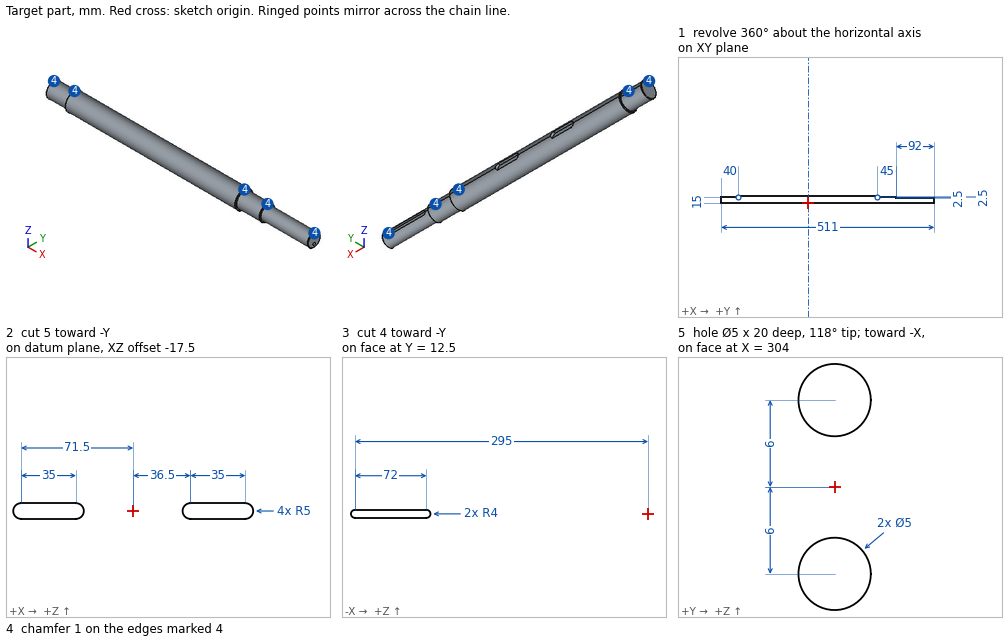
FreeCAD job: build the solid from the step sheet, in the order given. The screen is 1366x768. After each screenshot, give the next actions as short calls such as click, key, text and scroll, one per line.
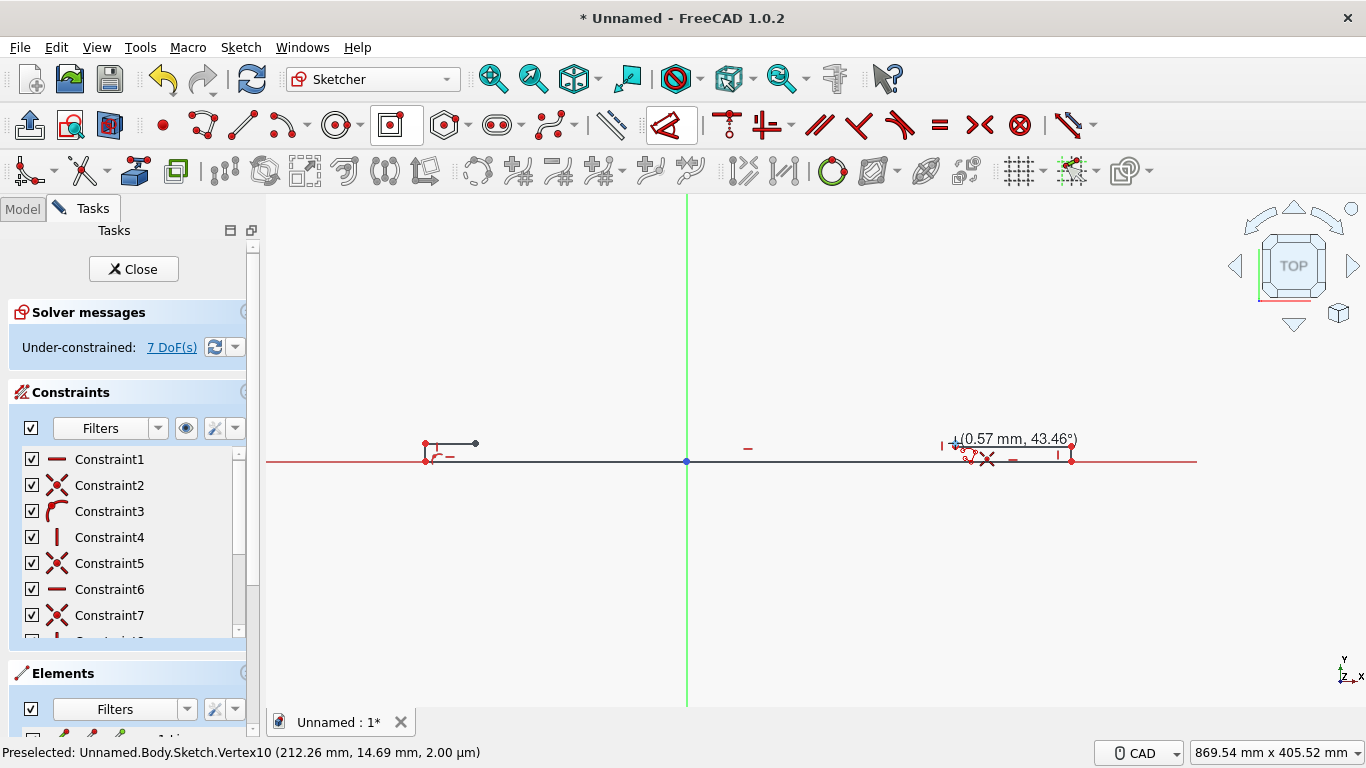
click(898, 443)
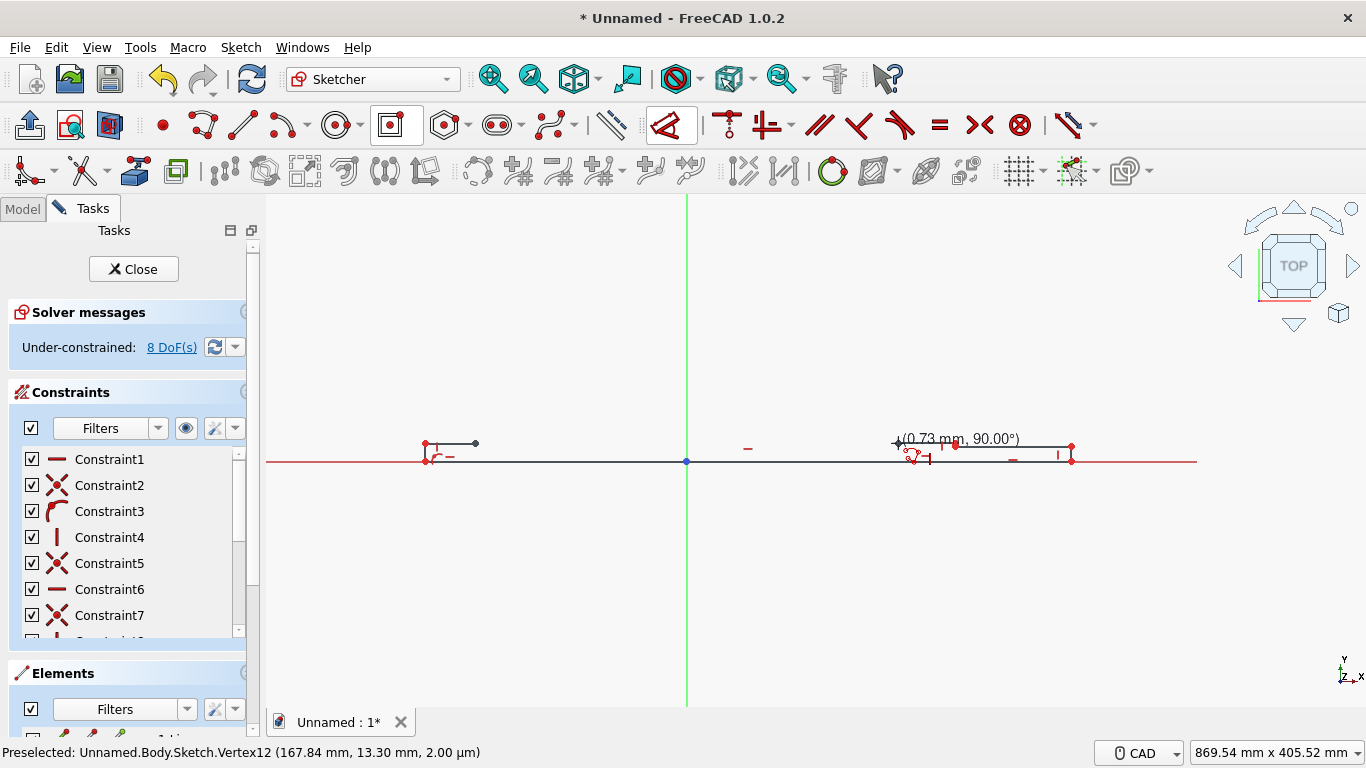
scroll(898, 440, up, 9)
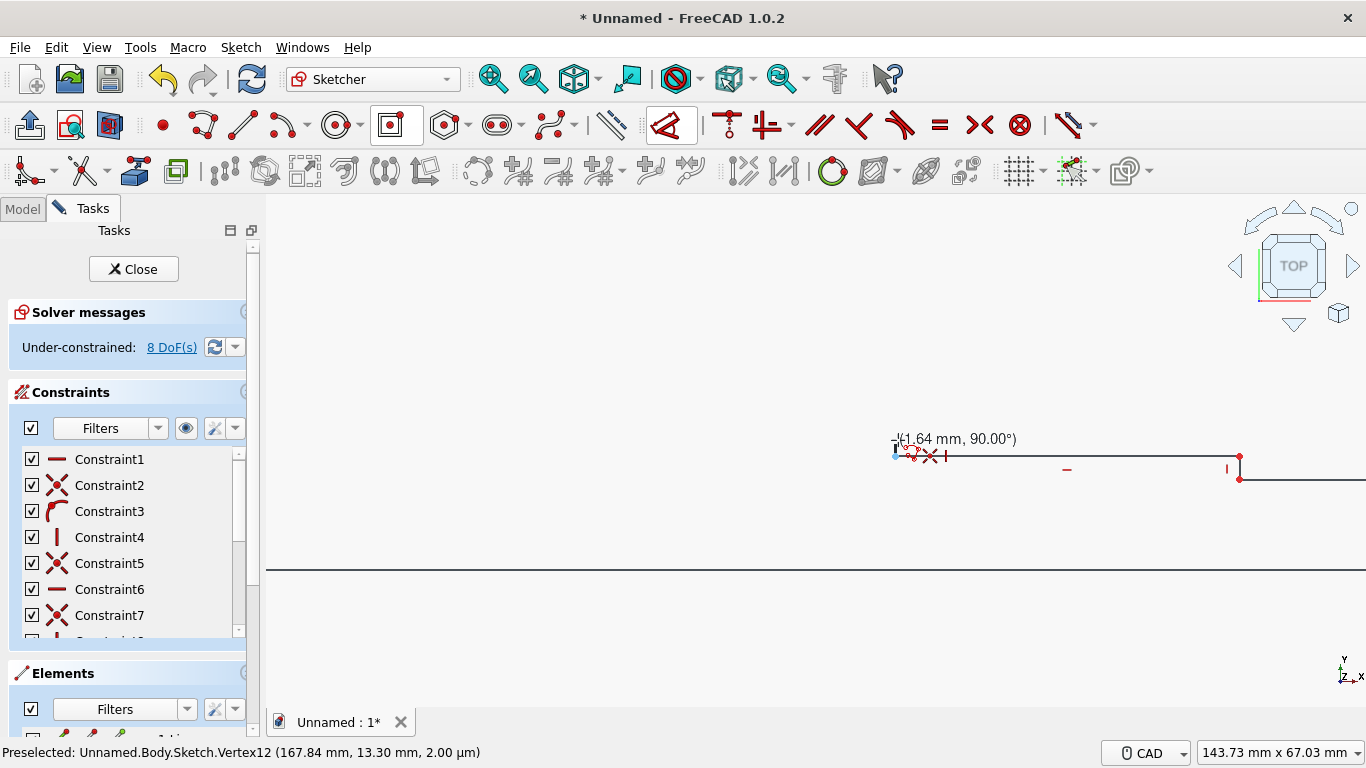
click(895, 436)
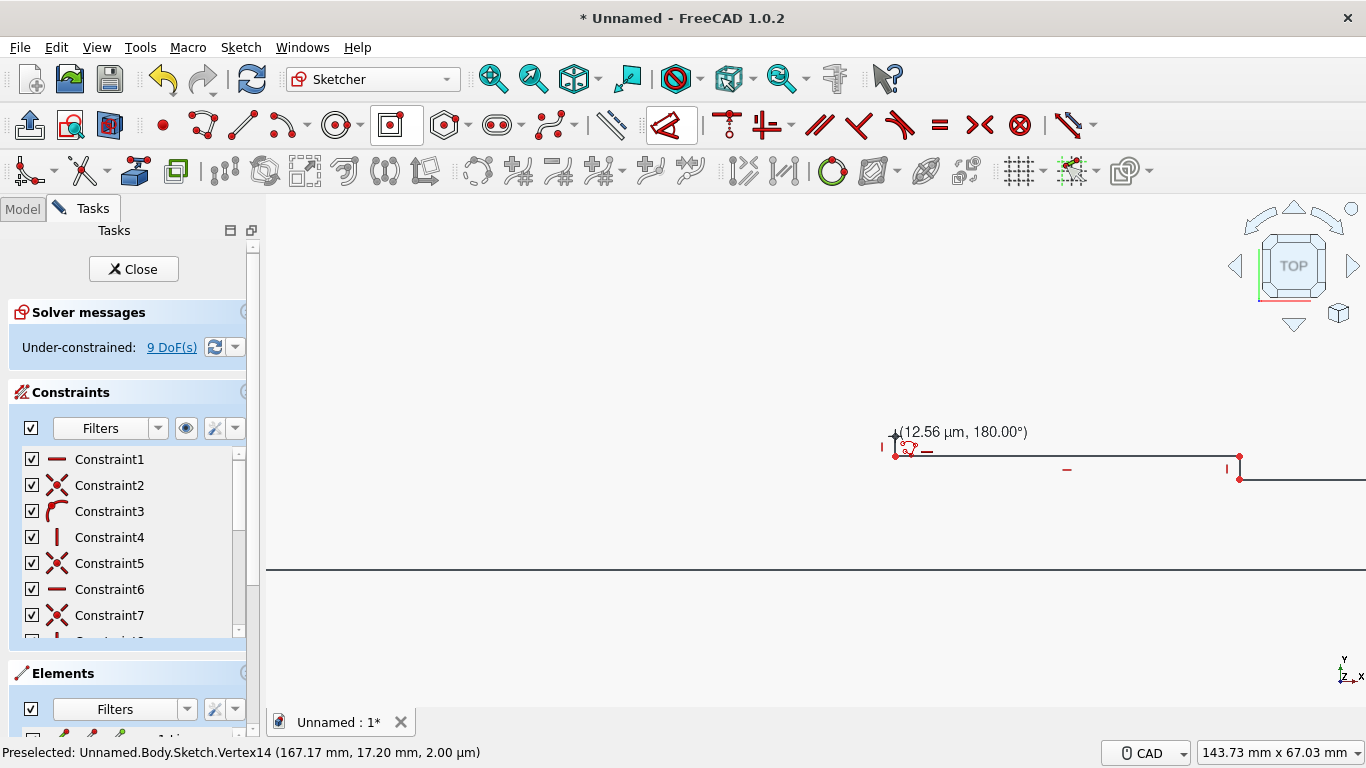
scroll(898, 440, down, 9)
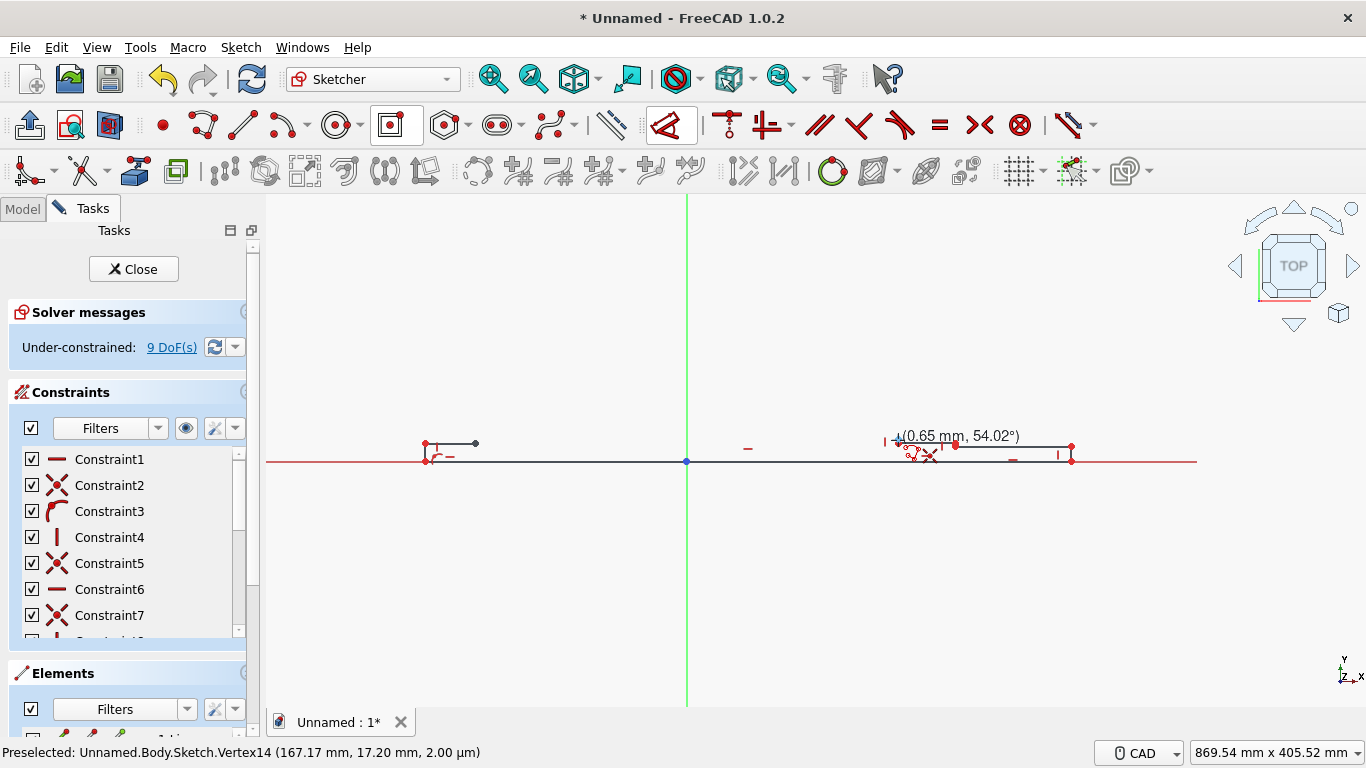
scroll(475, 440, up, 9)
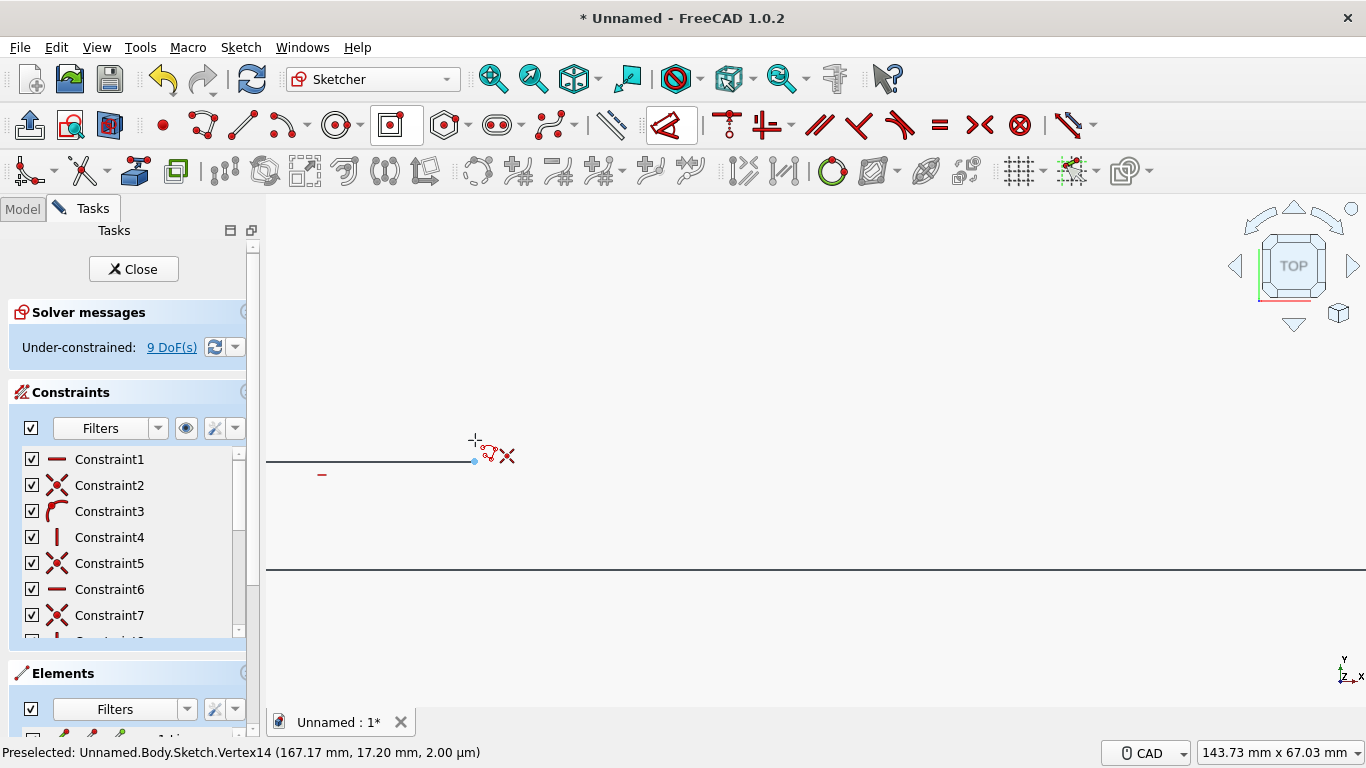
click(477, 436)
click(474, 462)
key(Escape)
key(Escape)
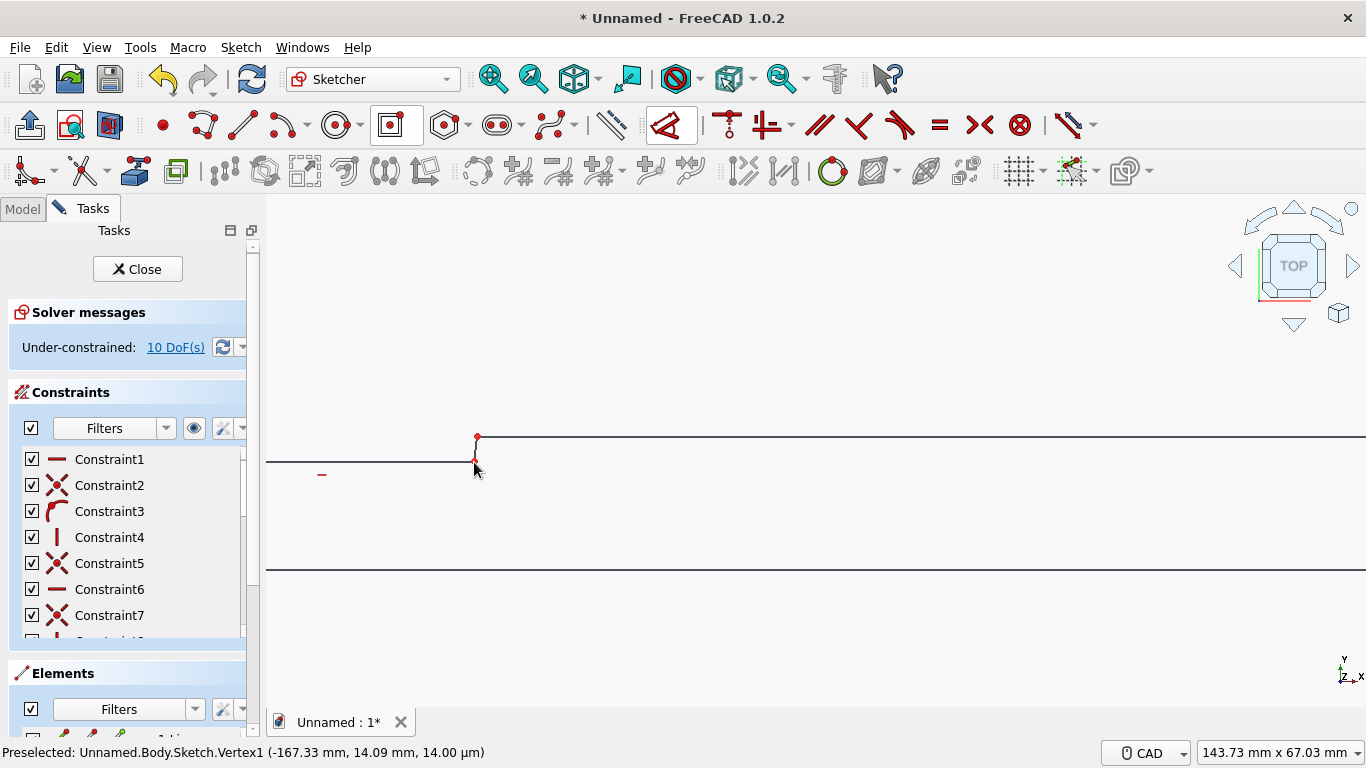
scroll(476, 447, up, 2)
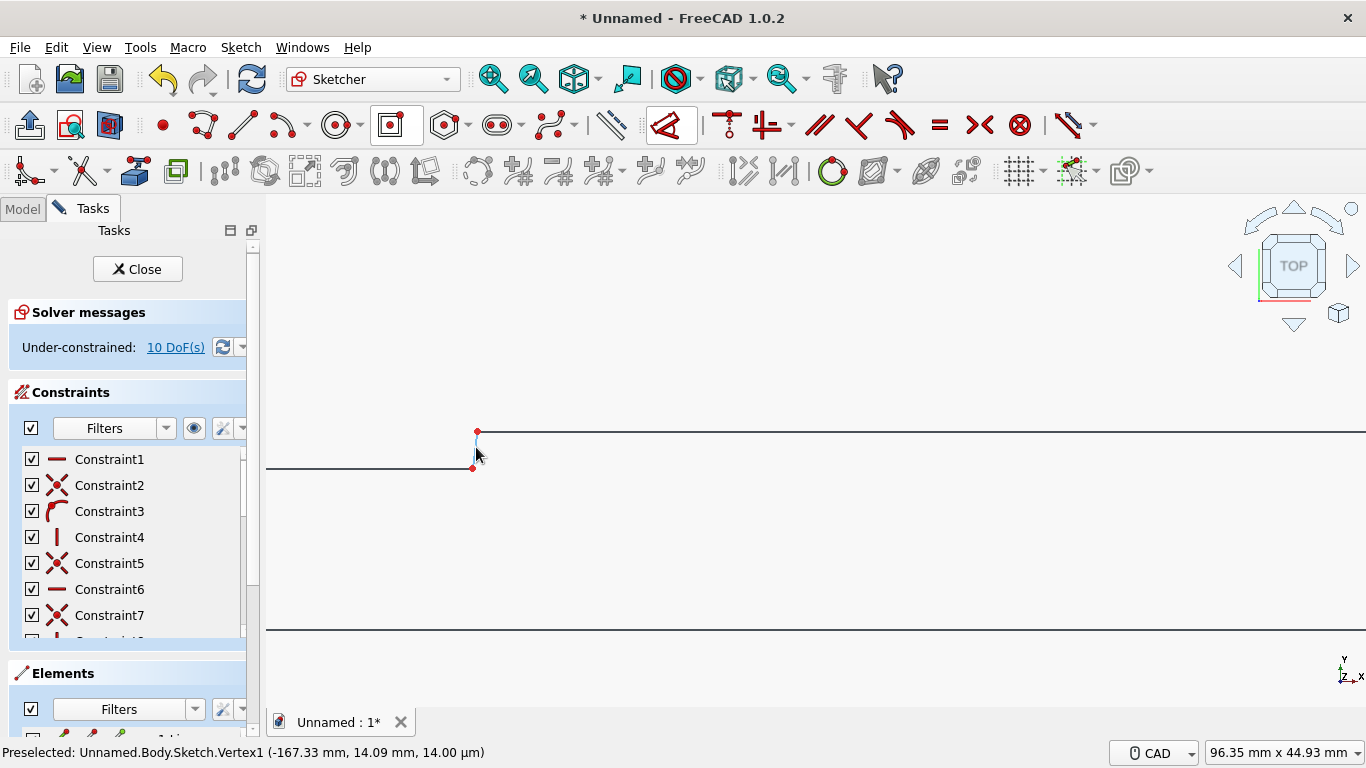
click(476, 447)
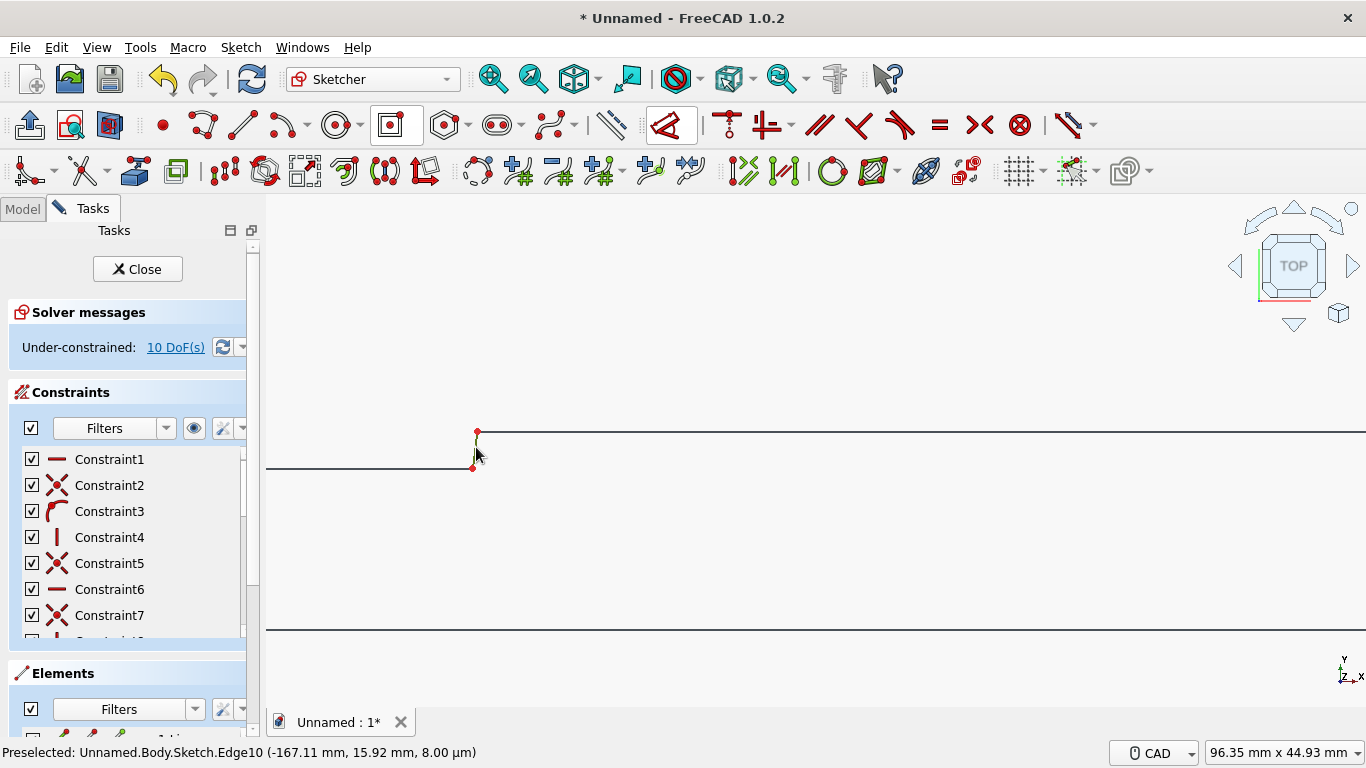
key(v)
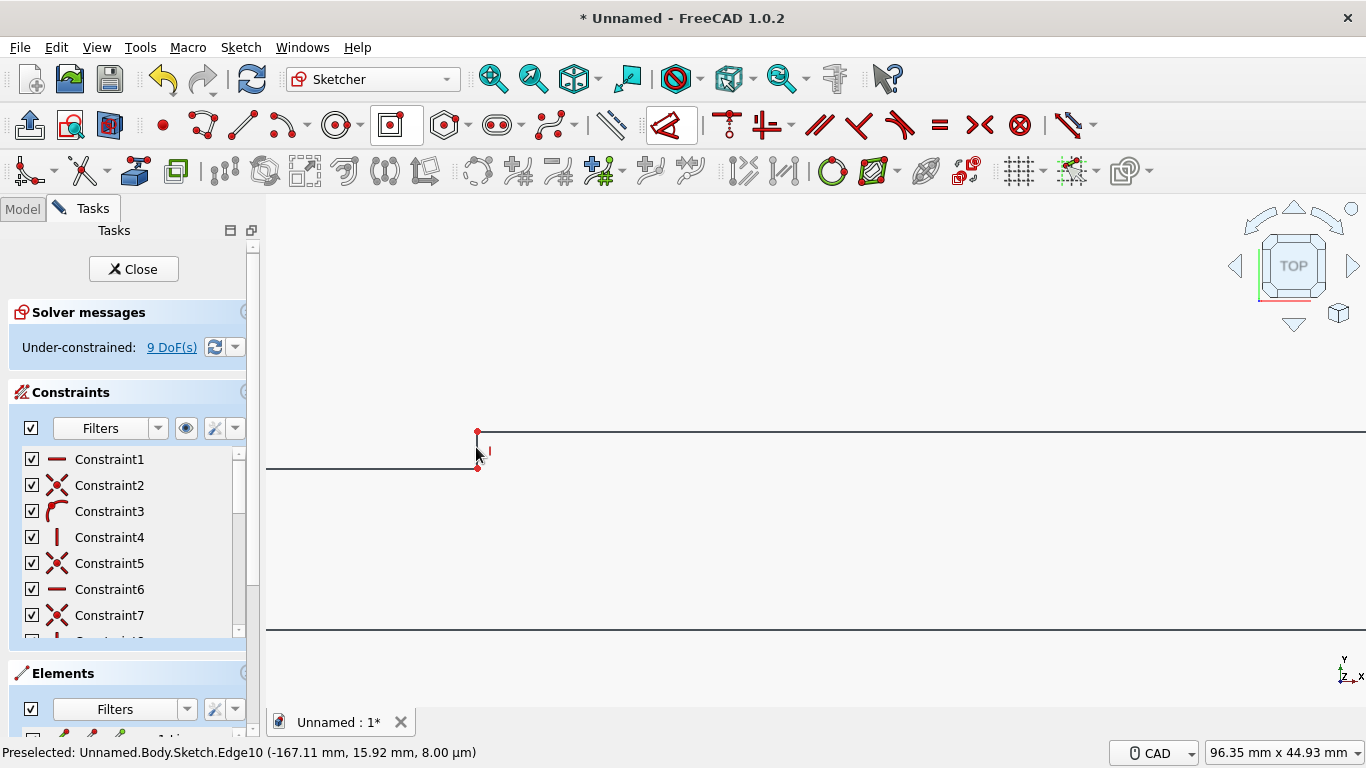
scroll(475, 441, down, 11)